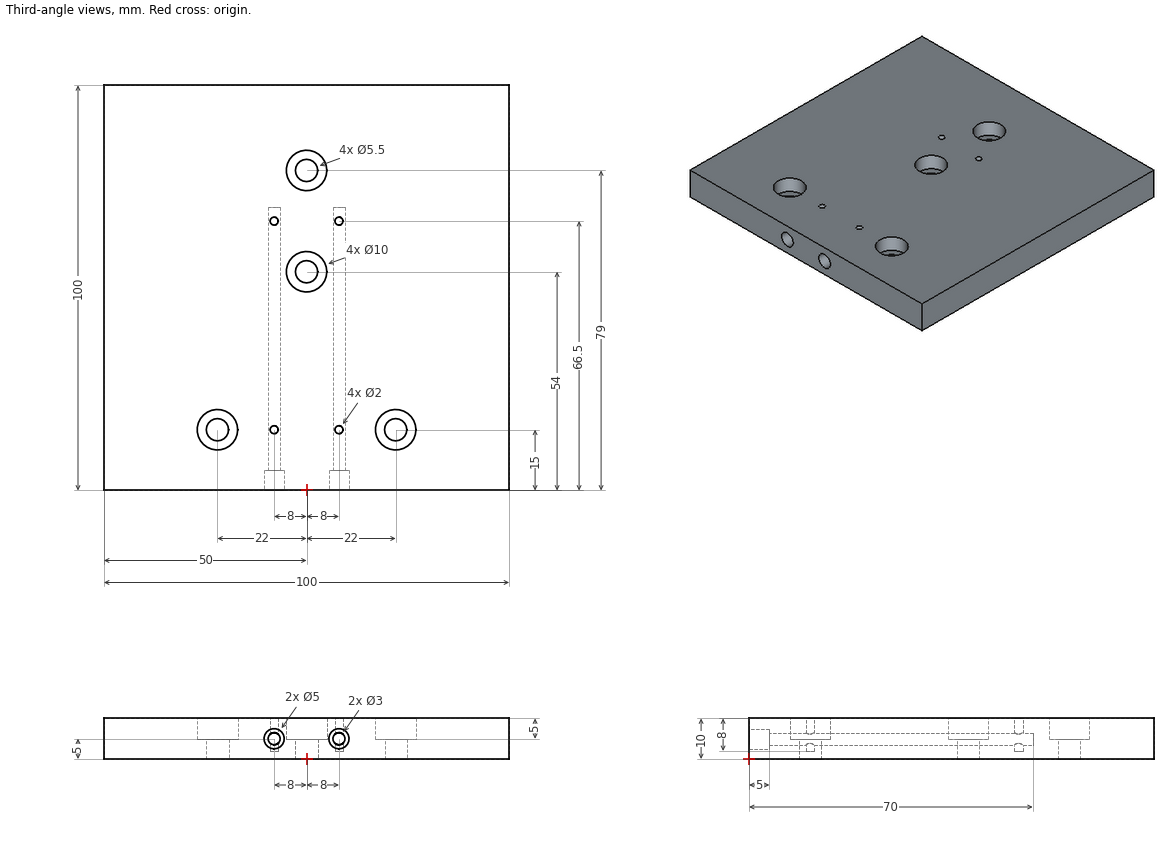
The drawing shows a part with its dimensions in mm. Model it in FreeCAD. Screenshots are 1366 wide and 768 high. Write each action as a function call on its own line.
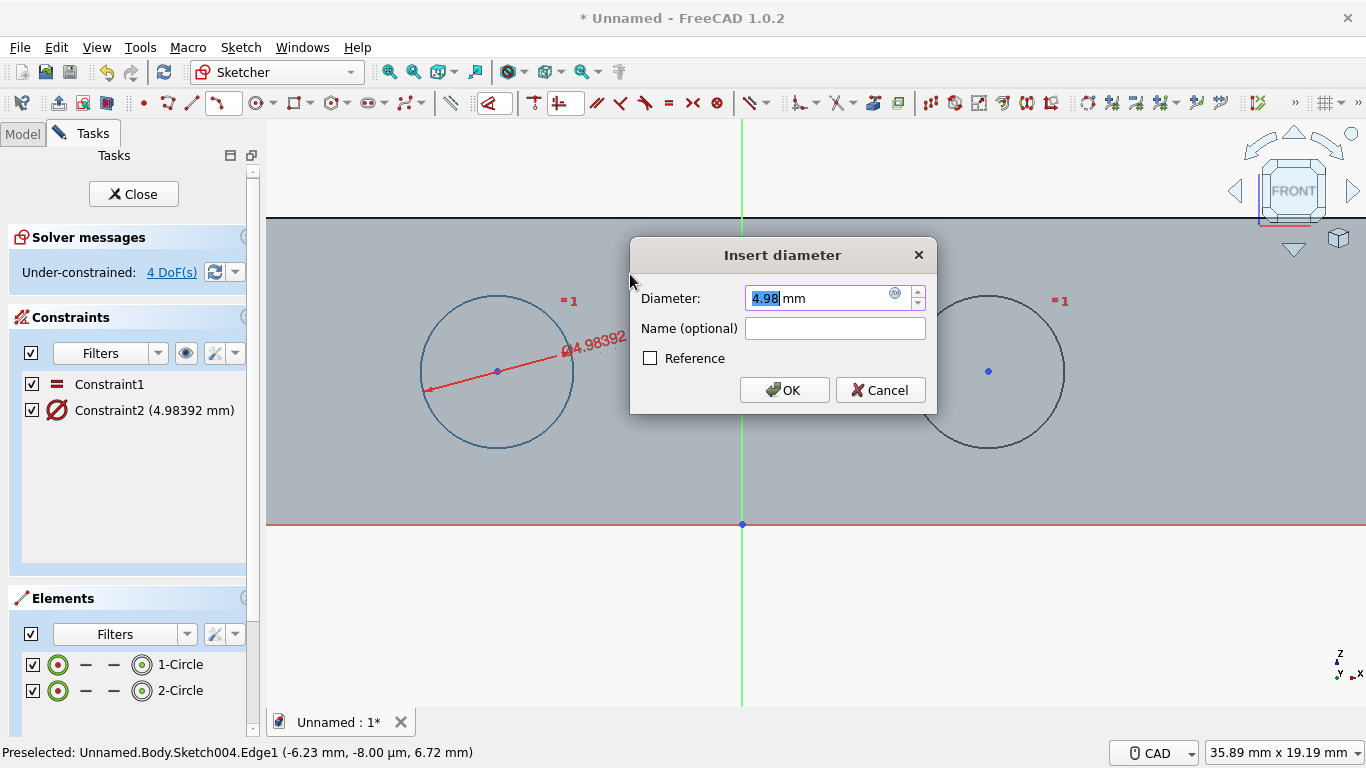
text(5)
key(Return)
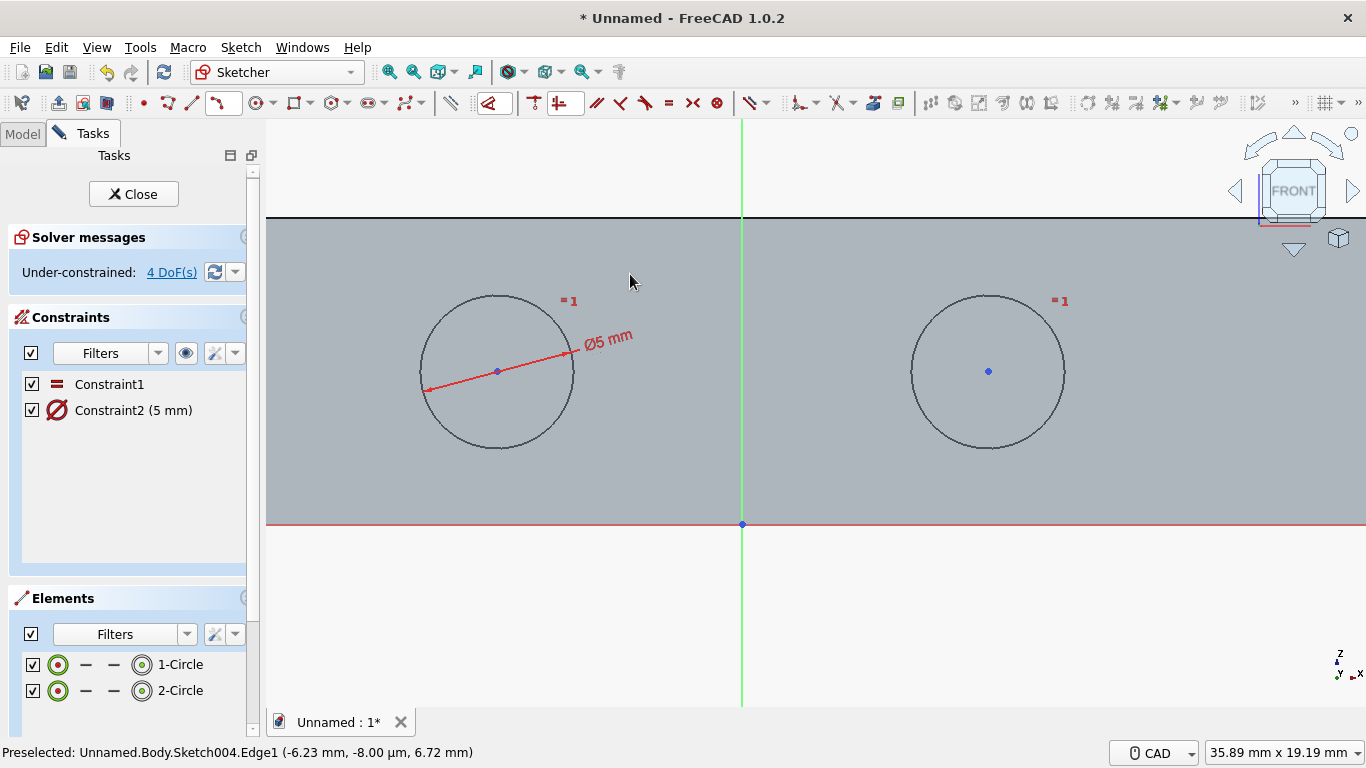
click(497, 372)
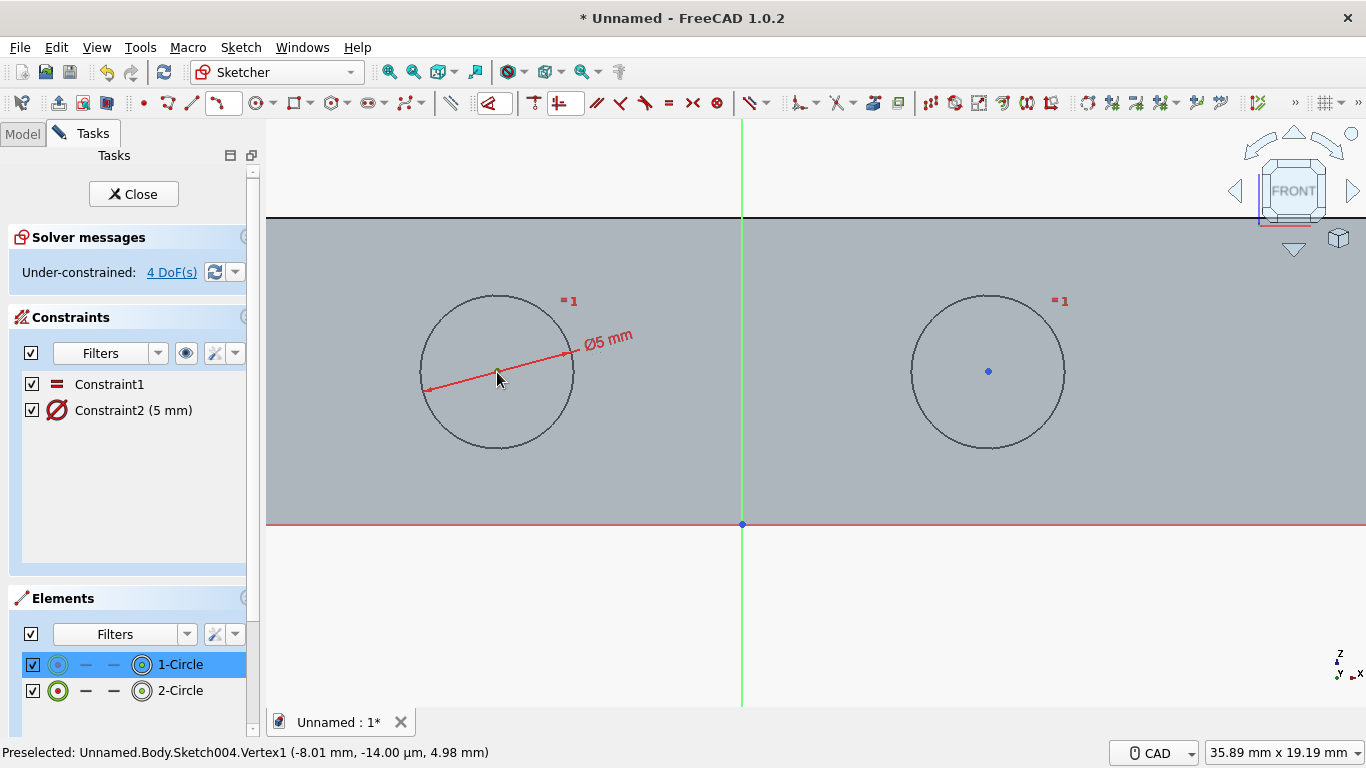
key(l)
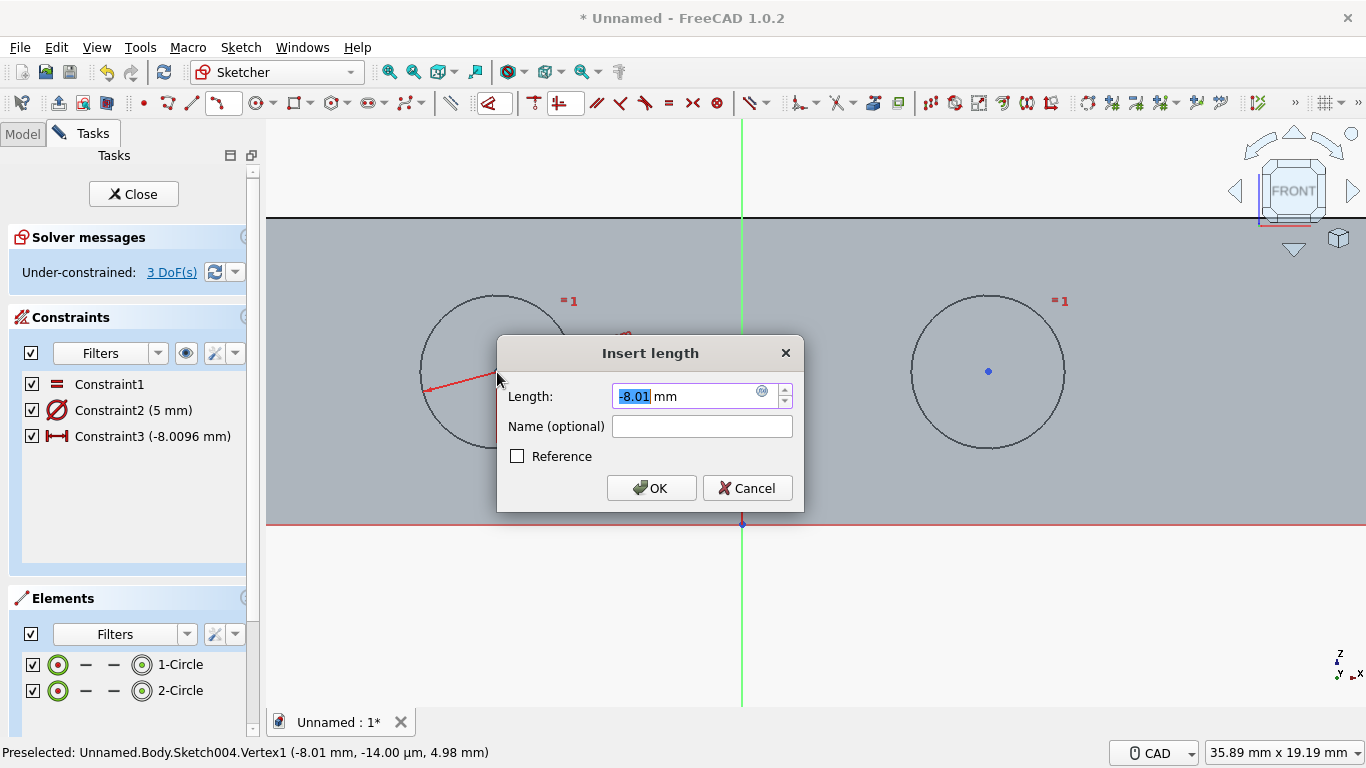
text(-8)
key(Return)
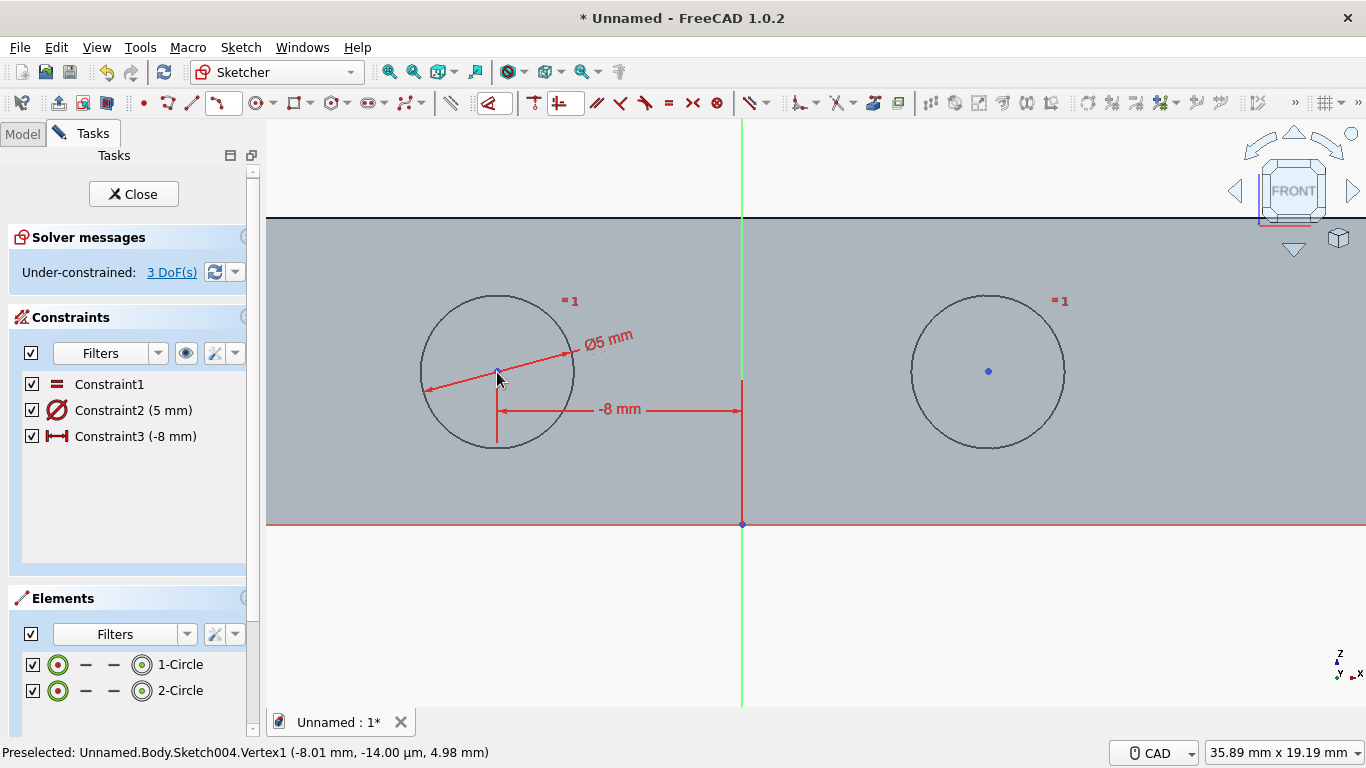
click(497, 372)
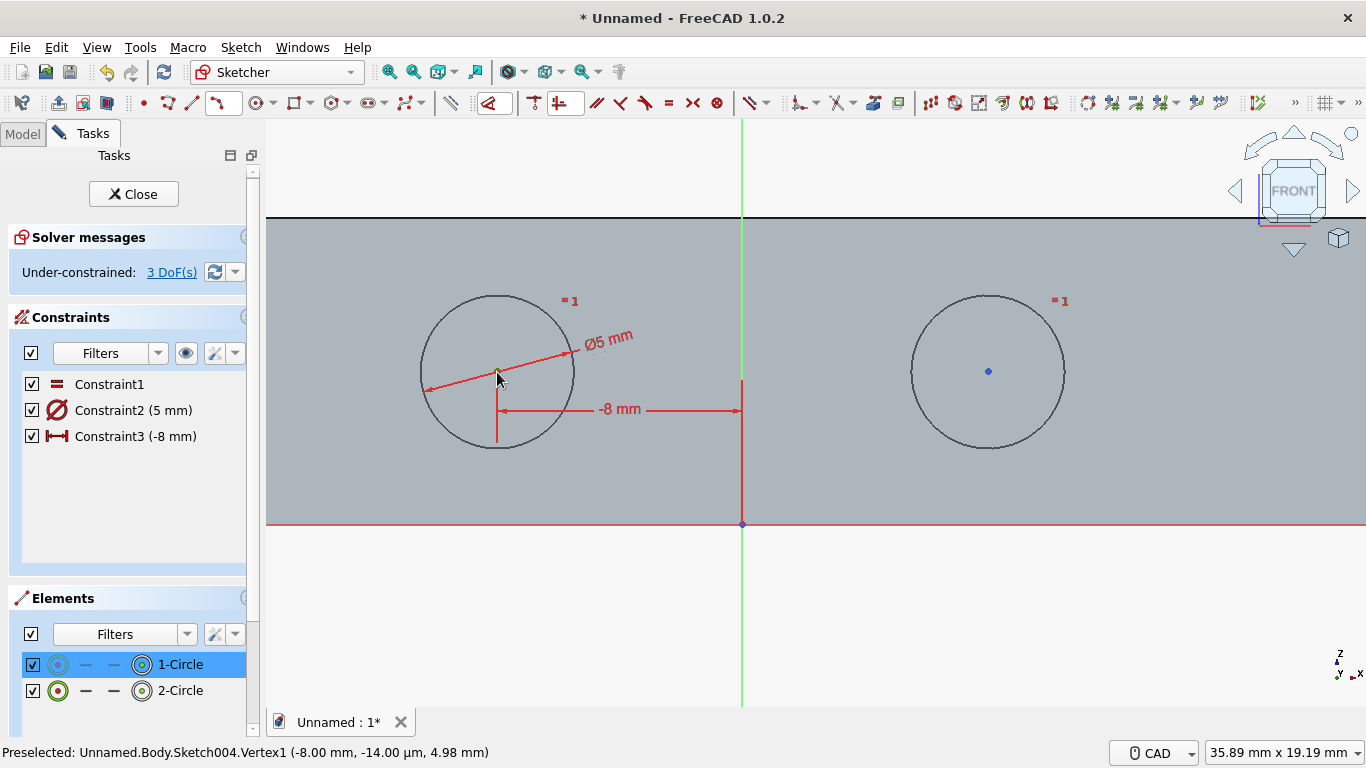
click(506, 104)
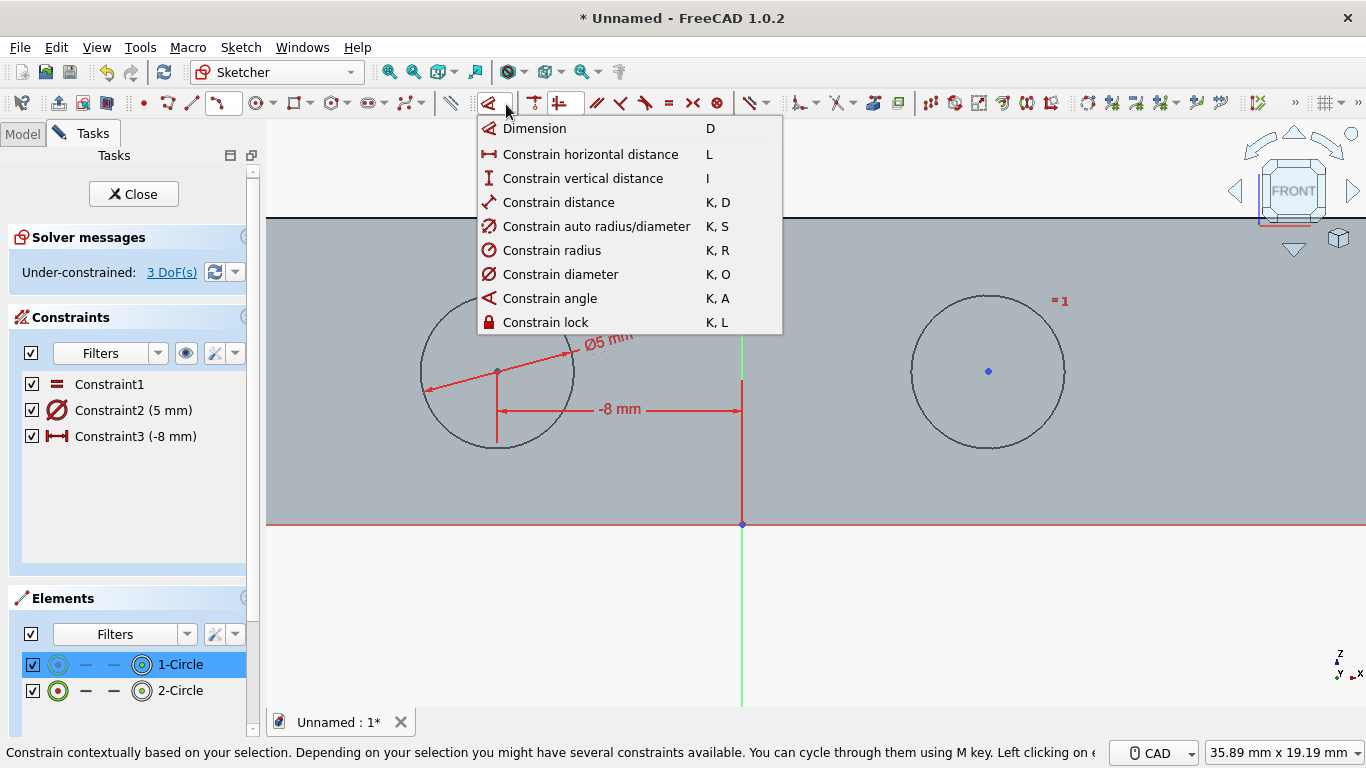
click(630, 178)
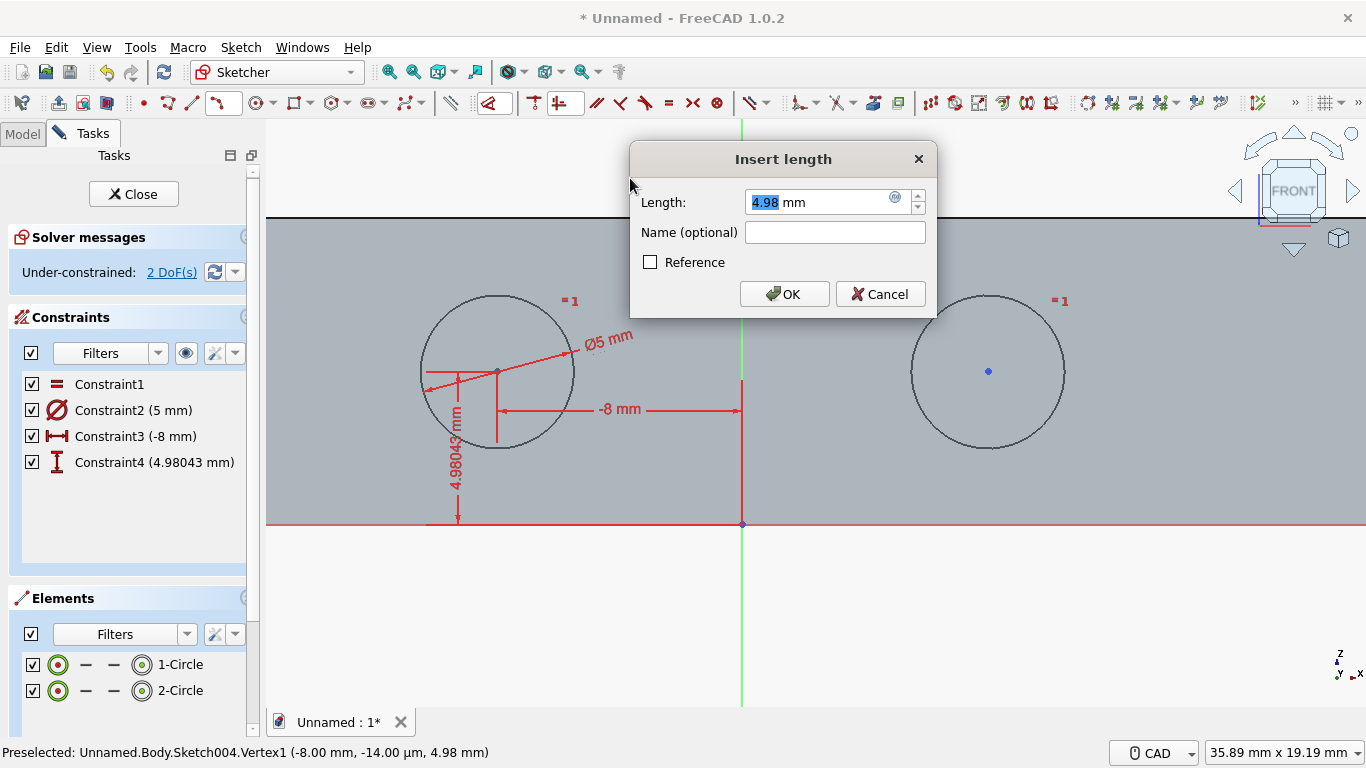
text(5)
key(Return)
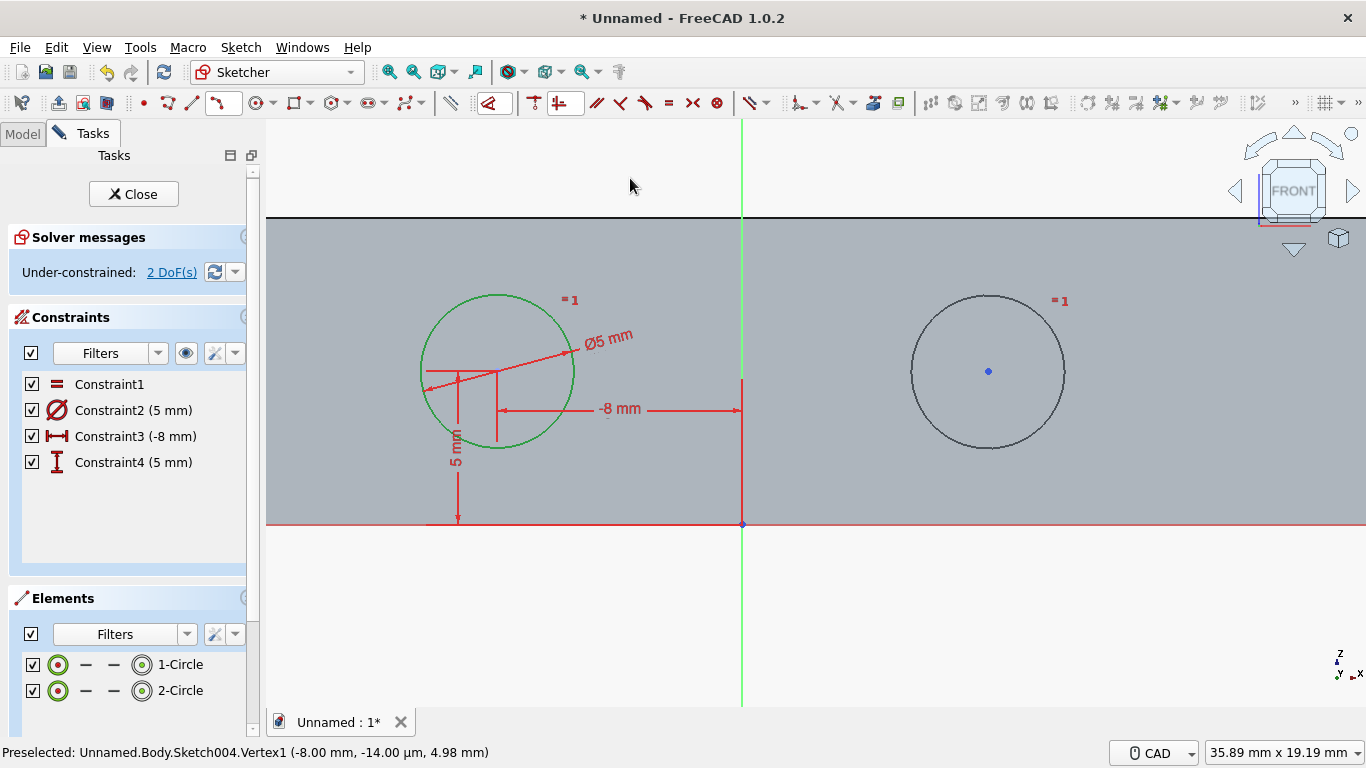
click(988, 372)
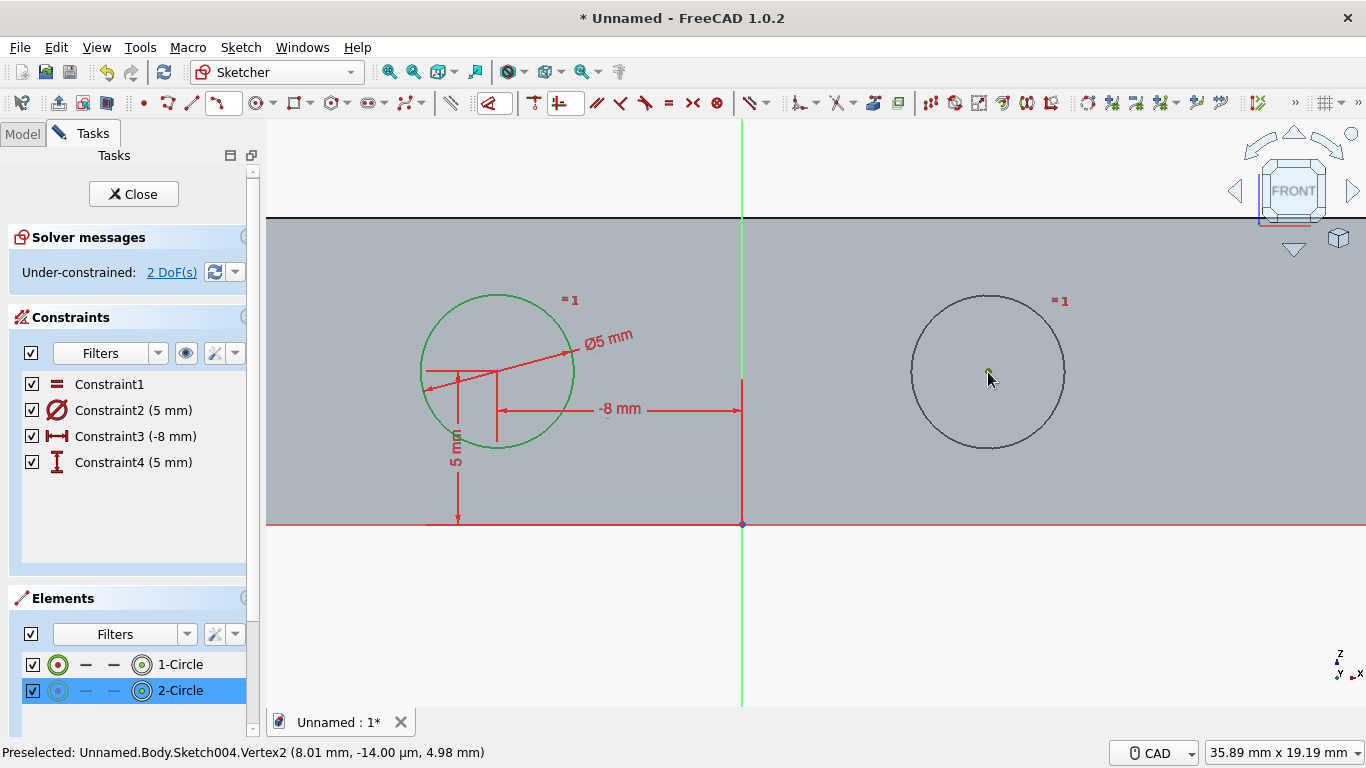
key(l)